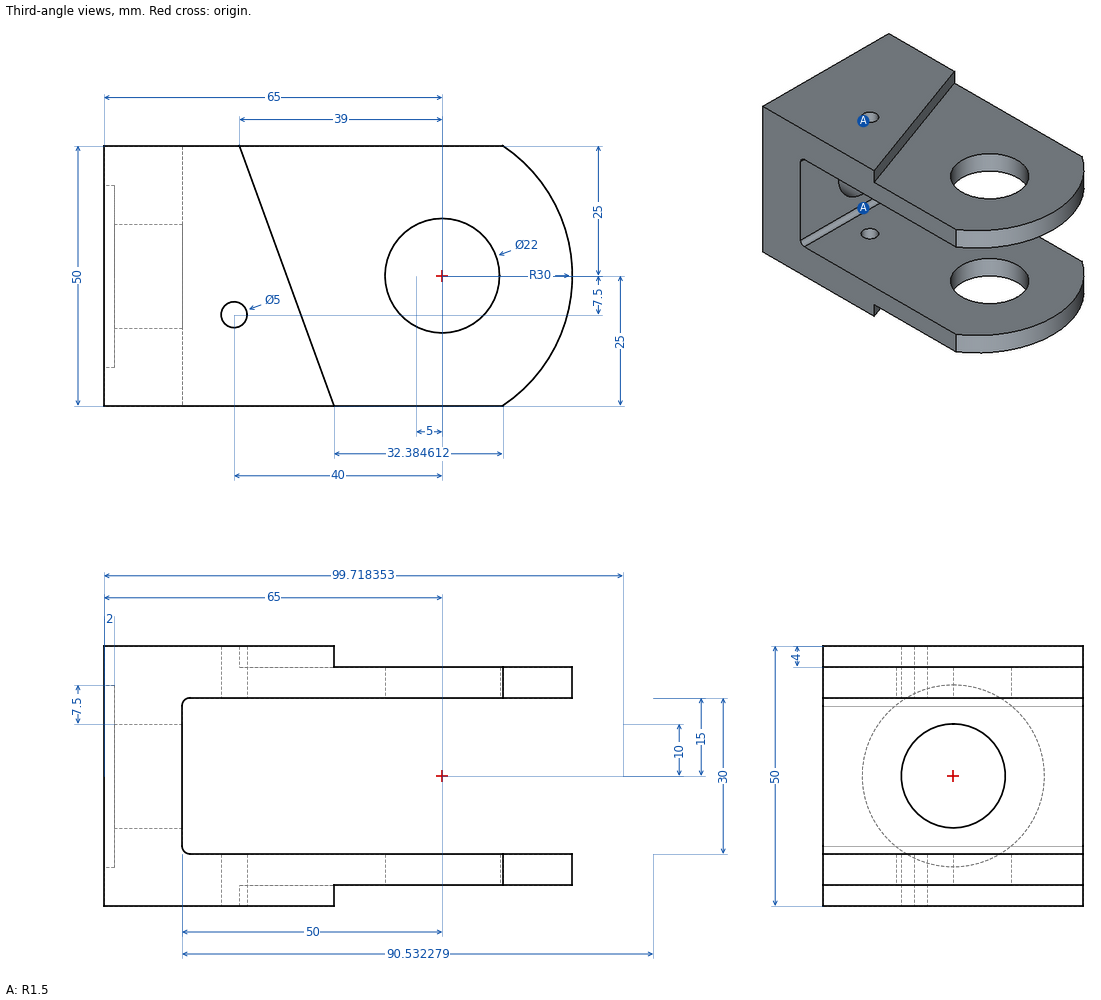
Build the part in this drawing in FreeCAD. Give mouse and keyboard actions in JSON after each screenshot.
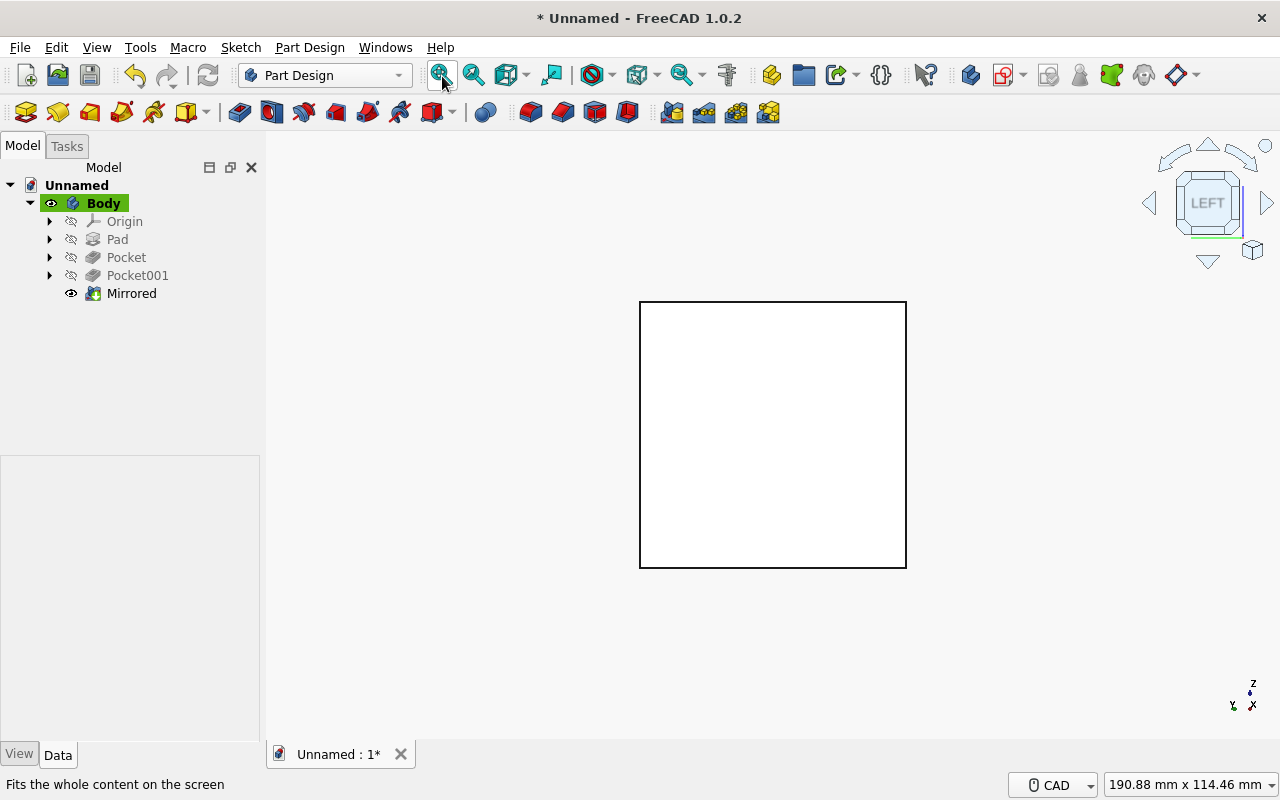
{"action": "key", "text": "v 3"}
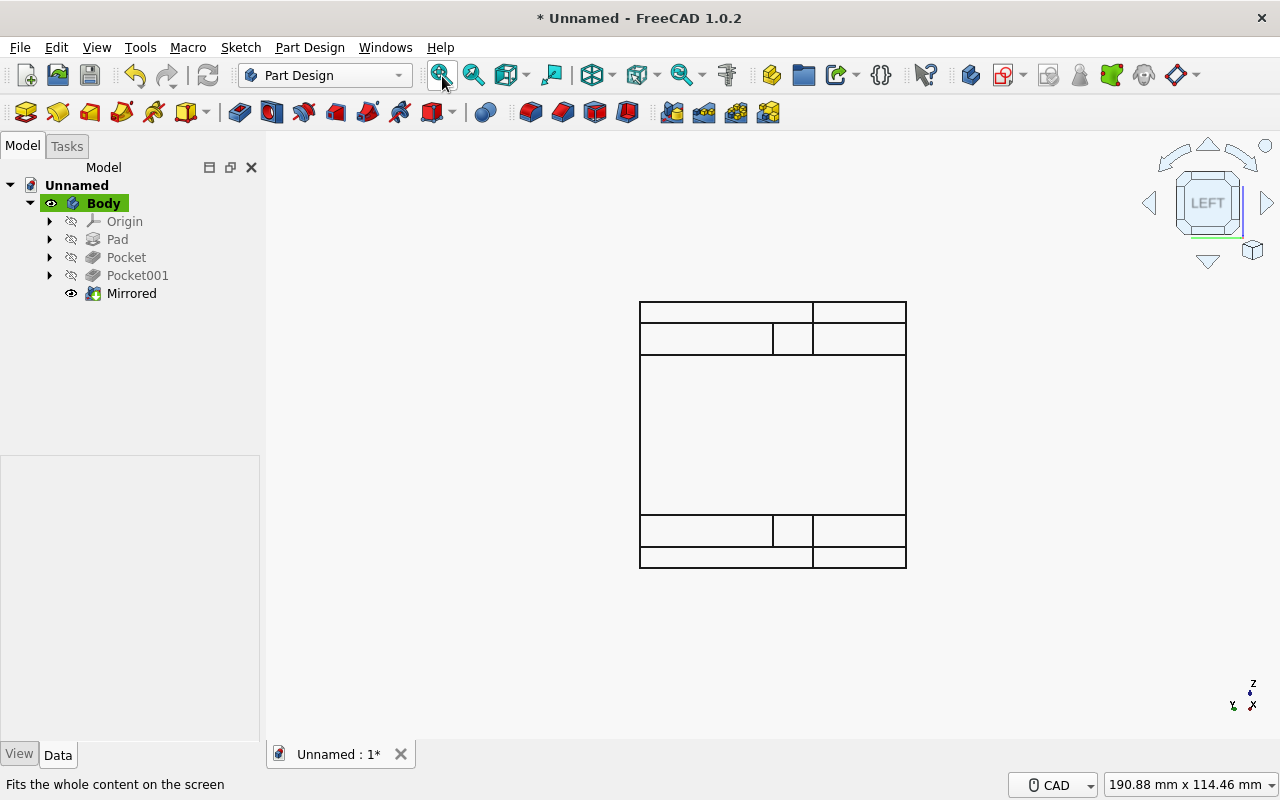
{"action": "key", "text": "0"}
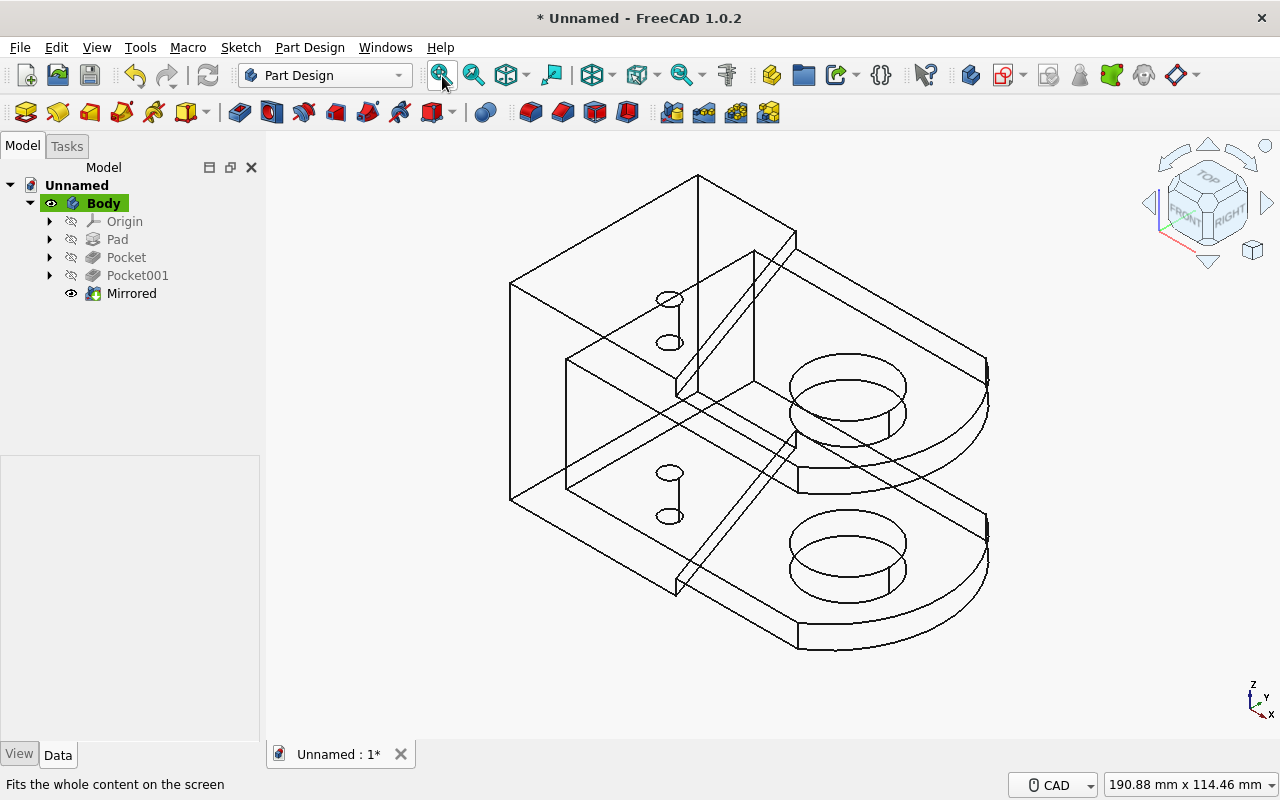
{"action": "left_click", "coordinate": [660, 434]}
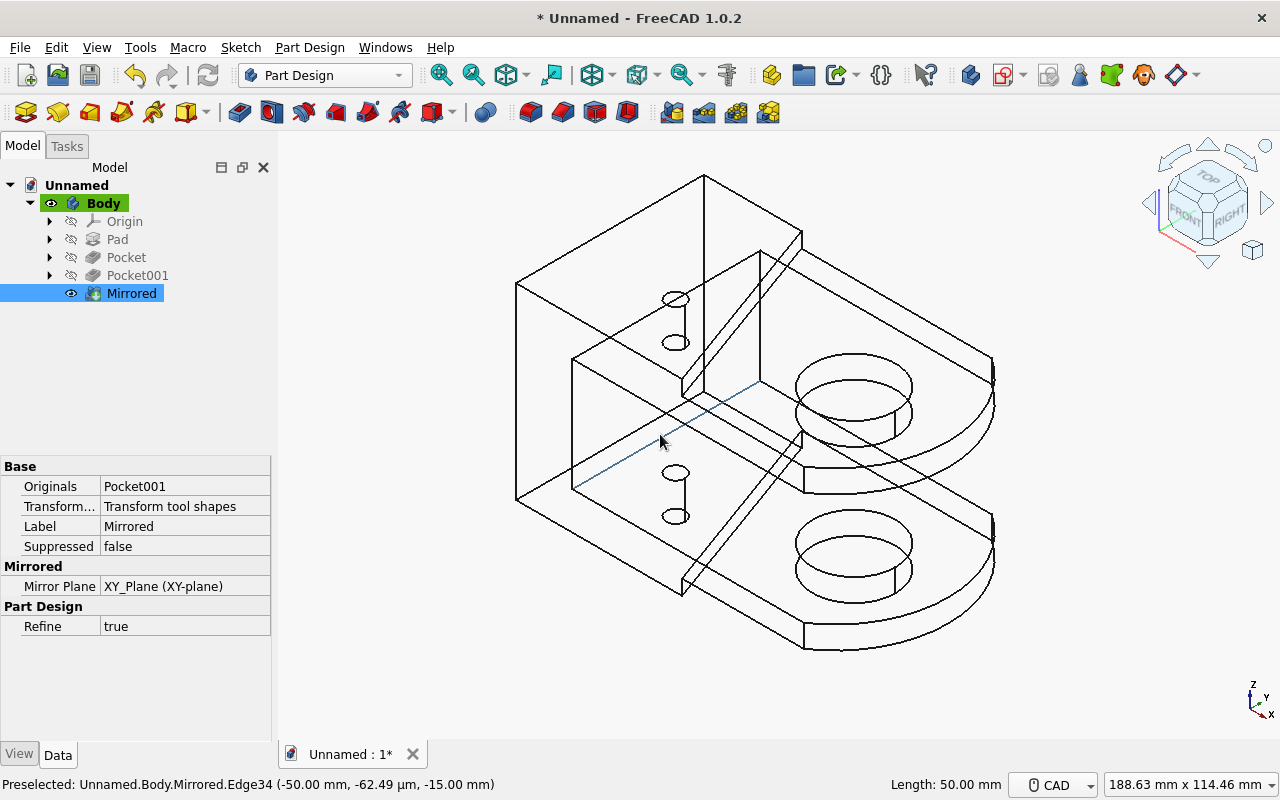
{"action": "left_click", "coordinate": [648, 315], "text": "ctrl"}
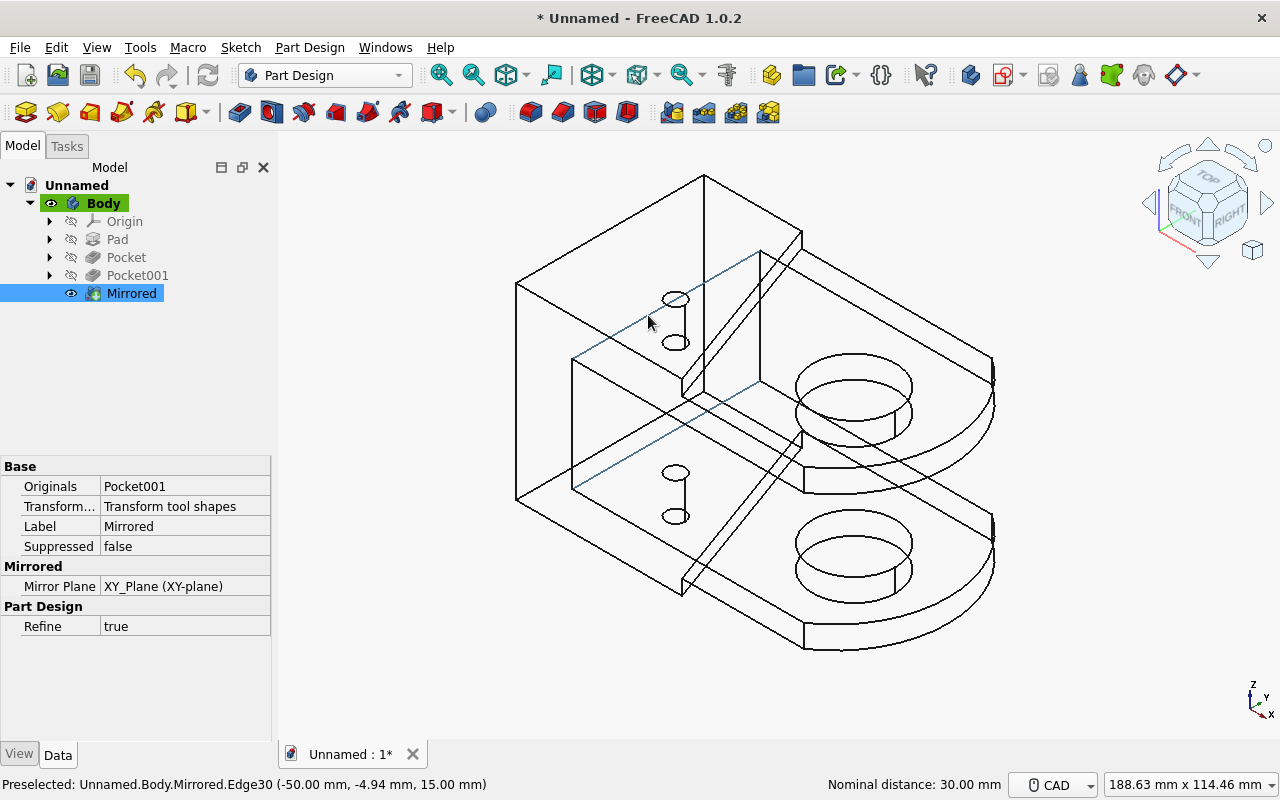
{"action": "key", "text": "v 1"}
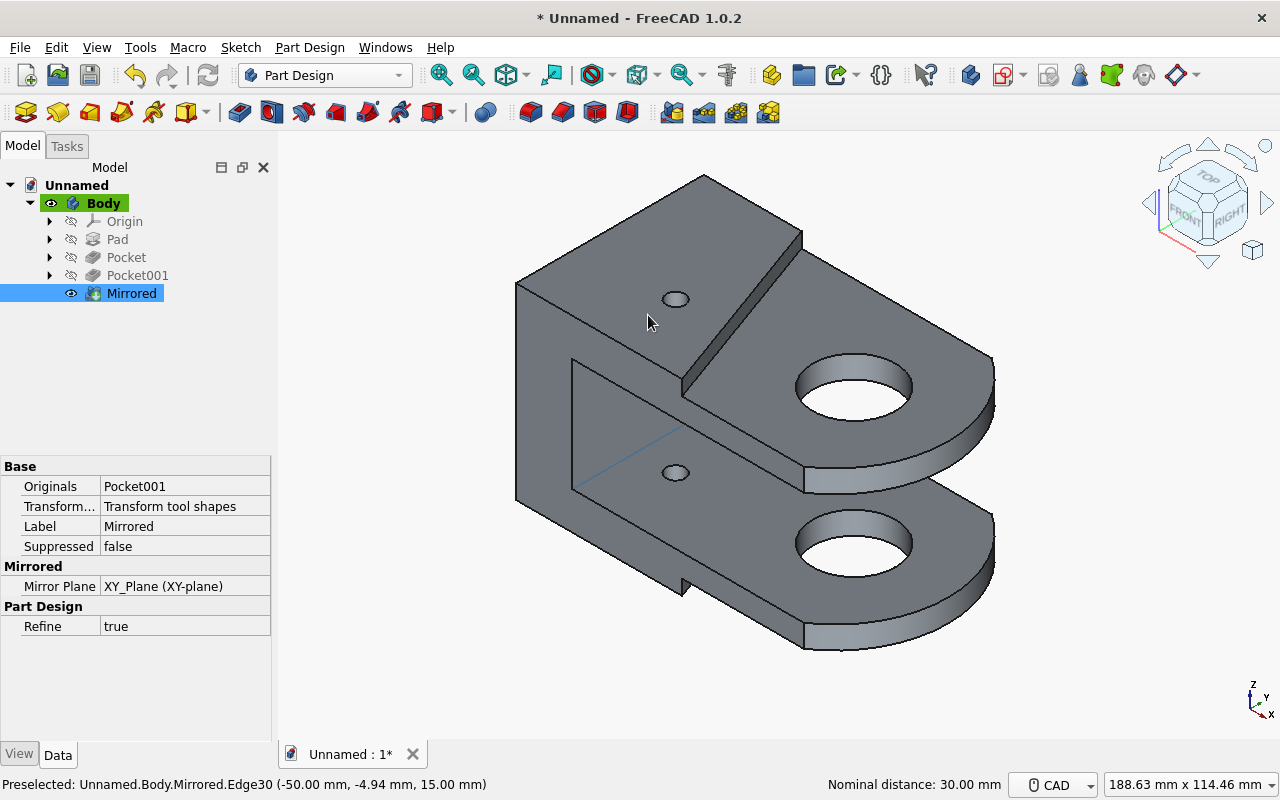
{"action": "left_click", "coordinate": [532, 112]}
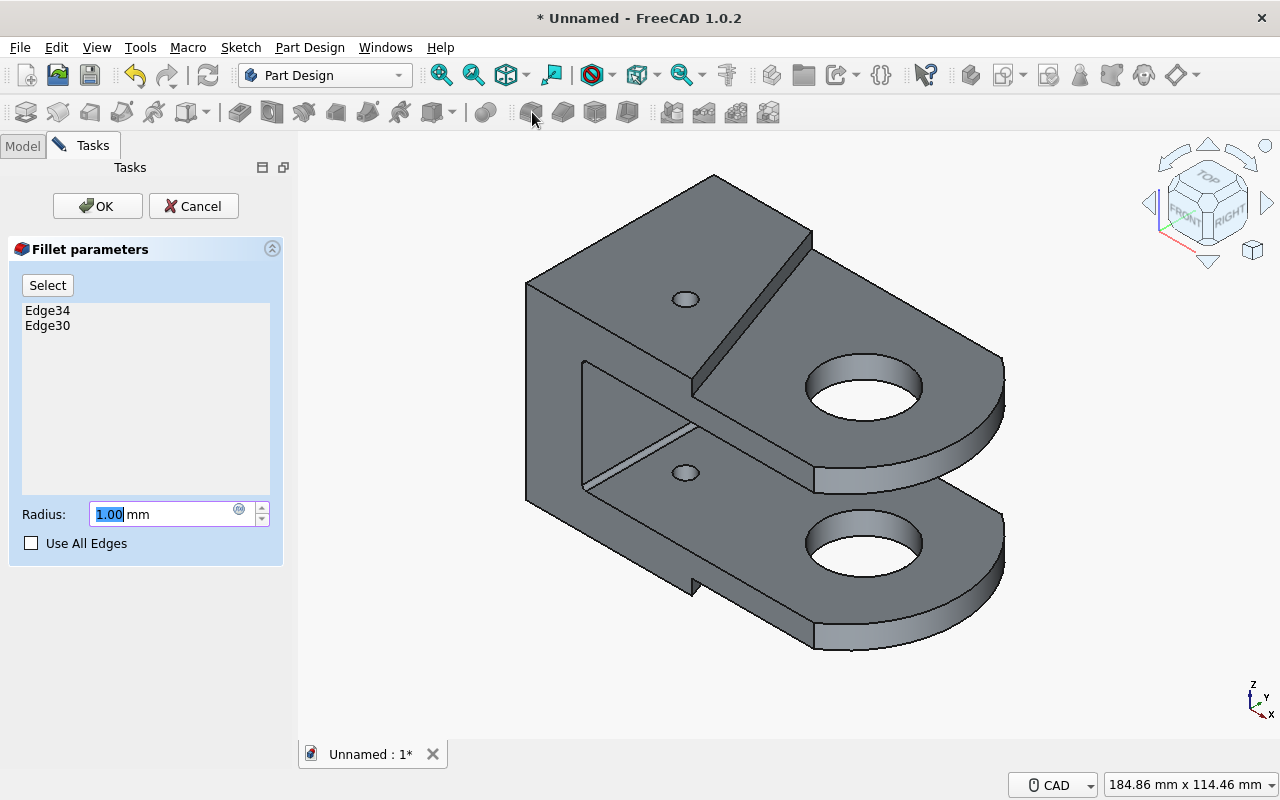
{"action": "type", "text": "1.5"}
{"action": "key", "text": "Tab"}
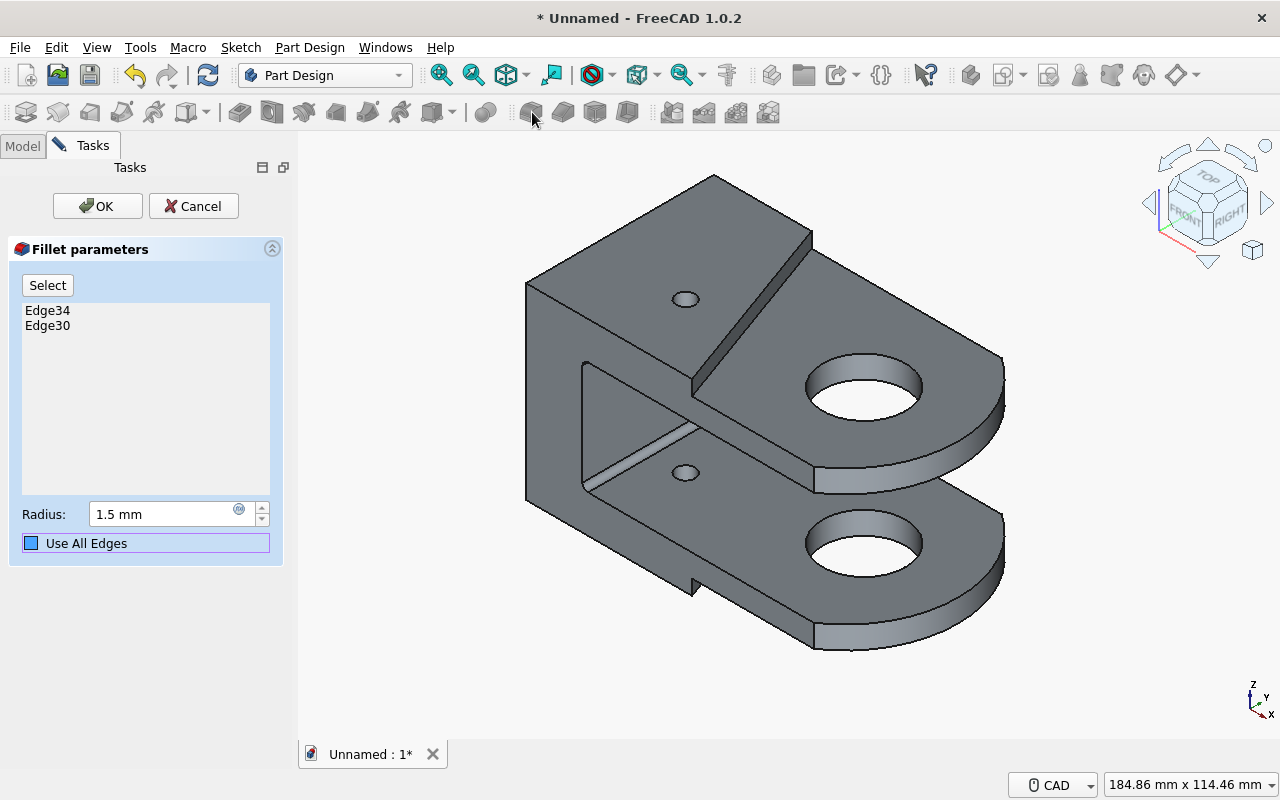
{"action": "left_click", "coordinate": [98, 206]}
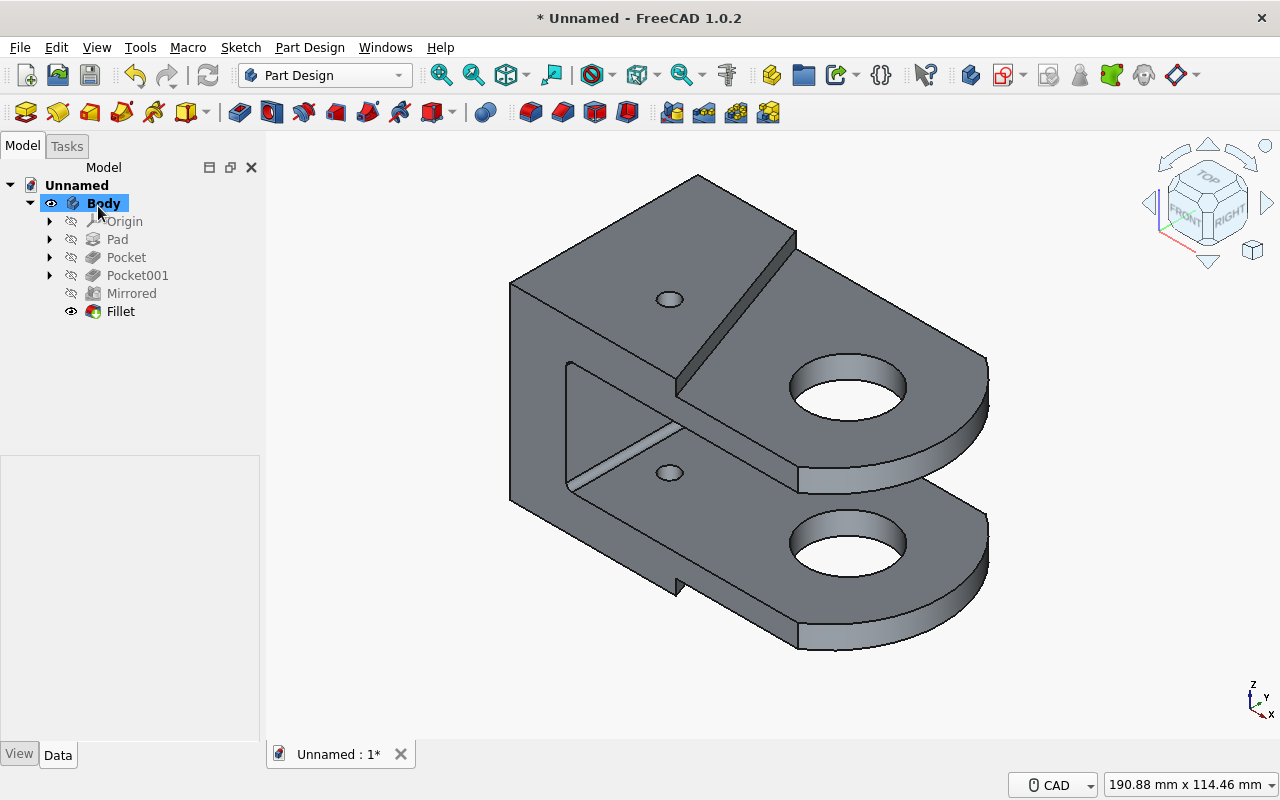
{"action": "left_click", "coordinate": [1004, 76]}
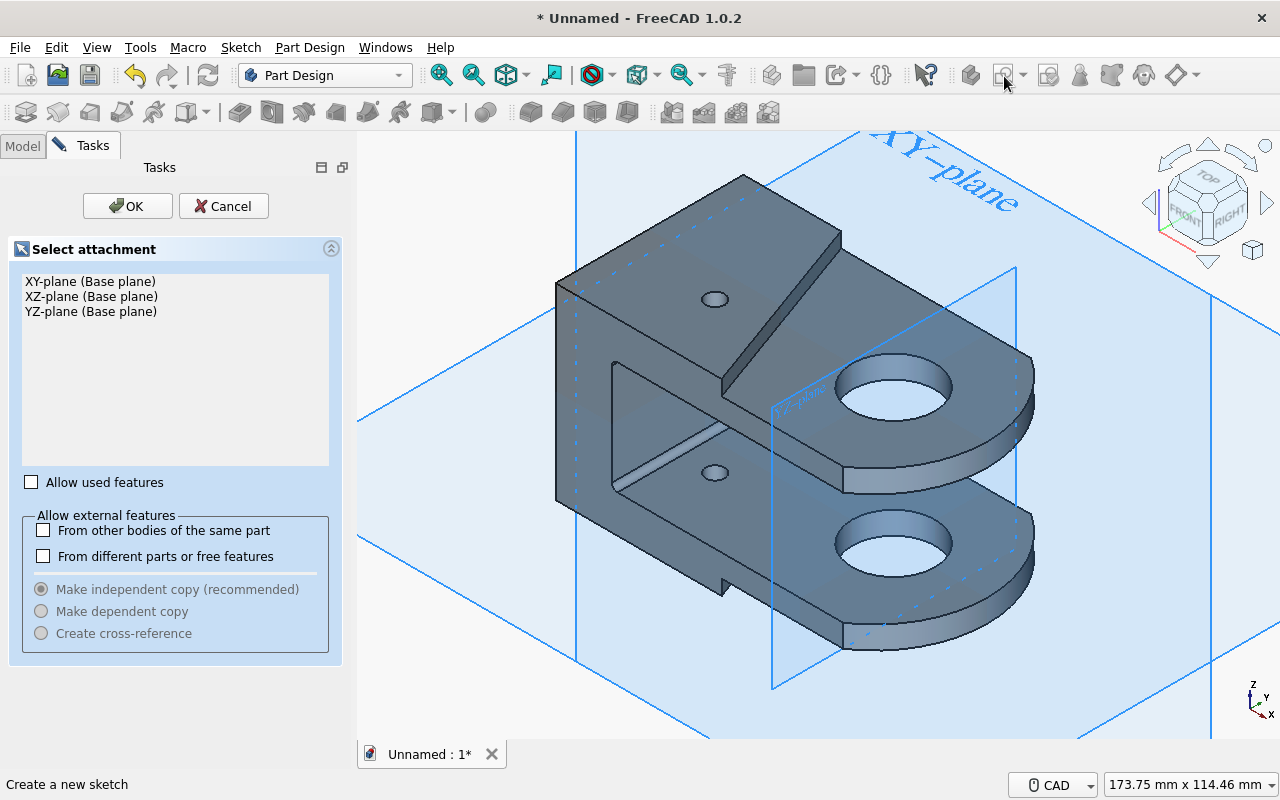
{"action": "left_click", "coordinate": [82, 296]}